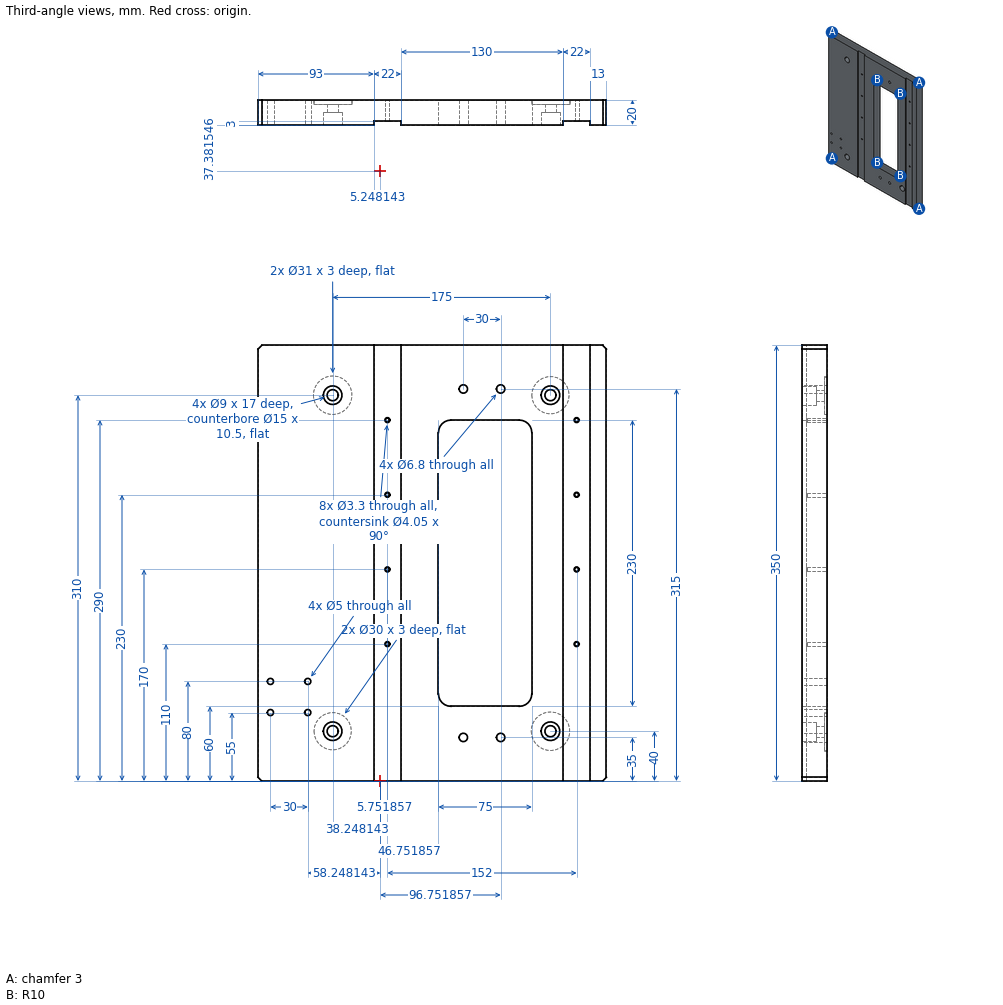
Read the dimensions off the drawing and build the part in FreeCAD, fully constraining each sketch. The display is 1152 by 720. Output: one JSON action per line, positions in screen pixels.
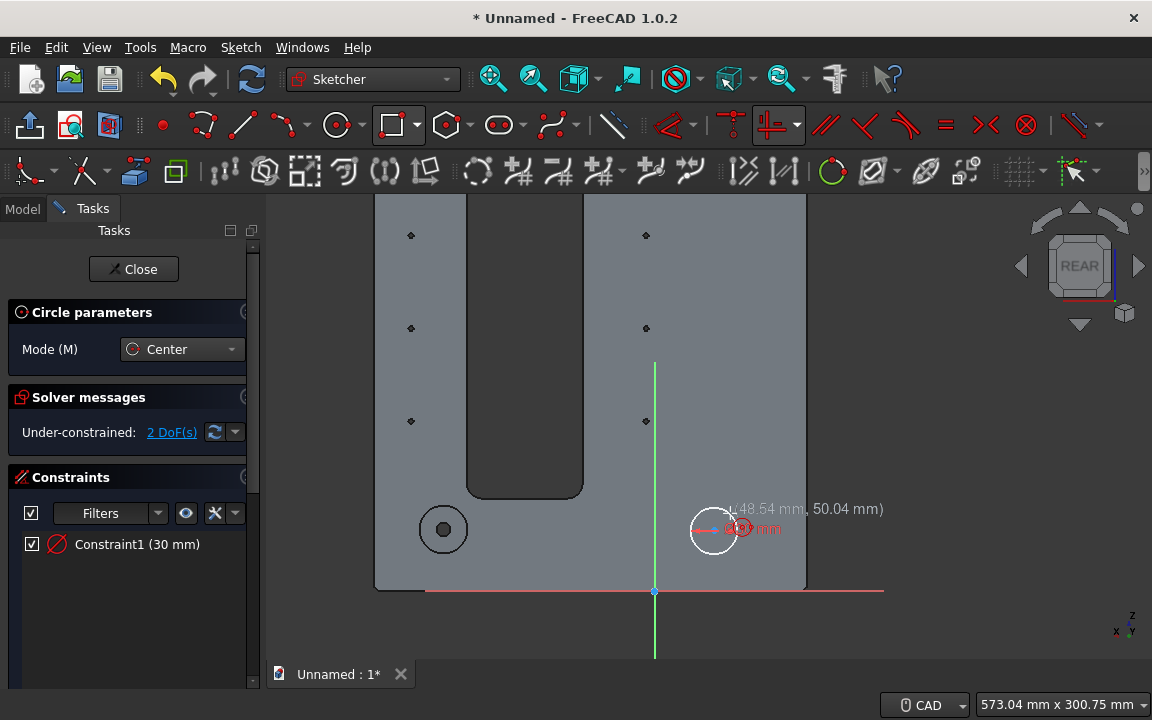
{"action": "scroll", "coordinate": [716, 532], "scroll_direction": "down", "scroll_amount": 3}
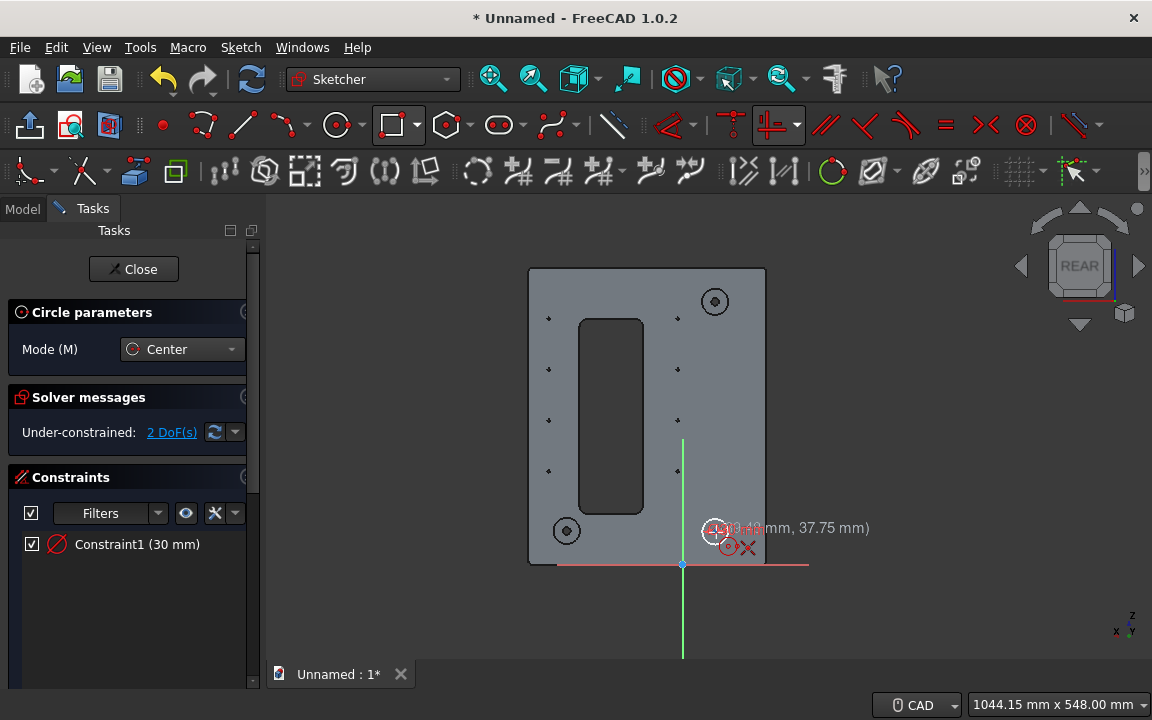
{"action": "scroll", "coordinate": [567, 302], "scroll_direction": "up", "scroll_amount": 3}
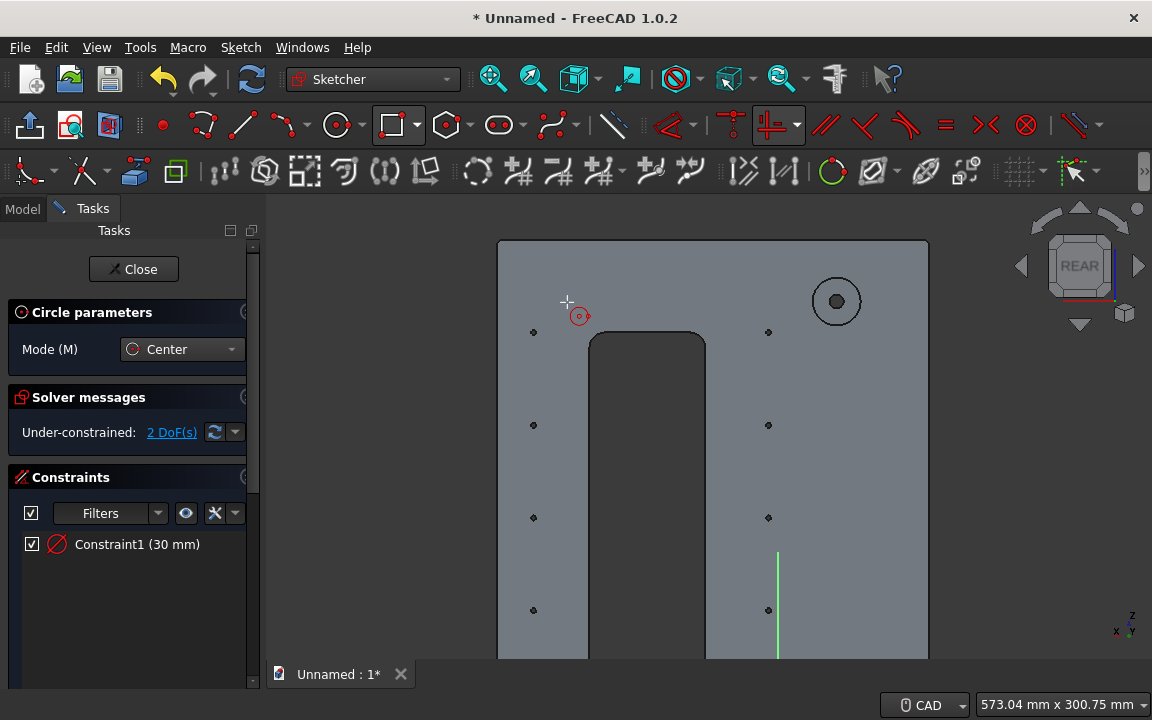
{"action": "left_click", "coordinate": [566, 302]}
{"action": "mouse_move", "coordinate": [583, 285]}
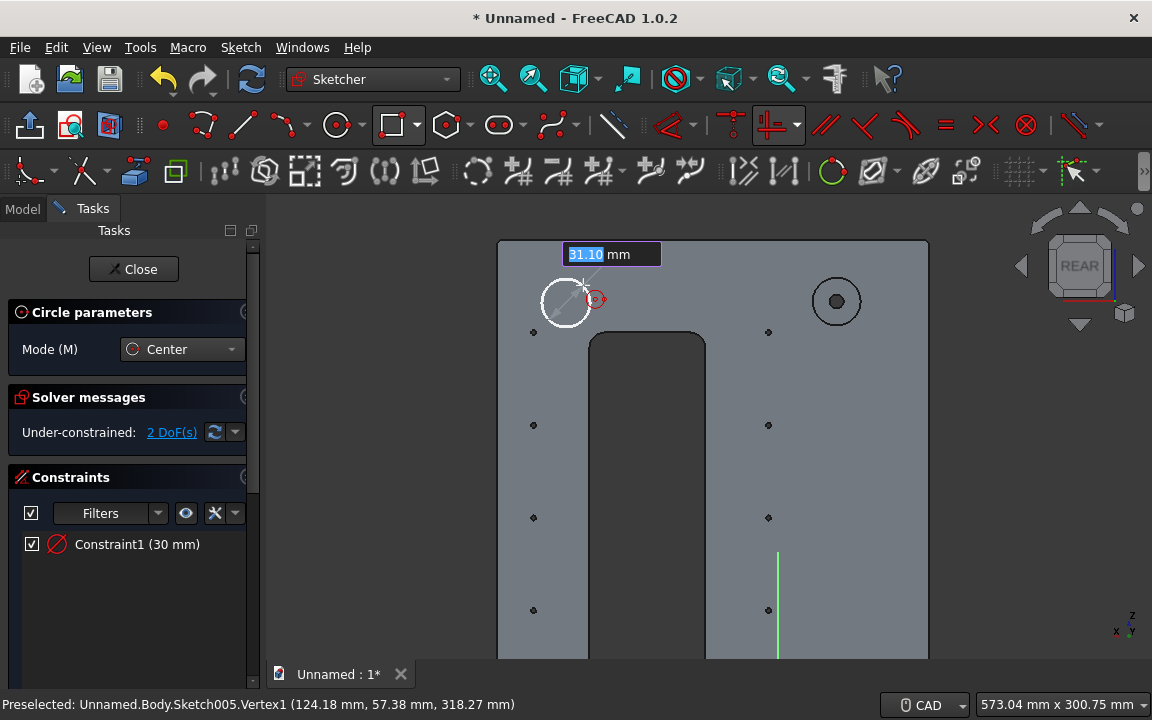
{"action": "type", "text": "30"}
{"action": "key", "text": "Return"}
{"action": "key", "text": "Escape"}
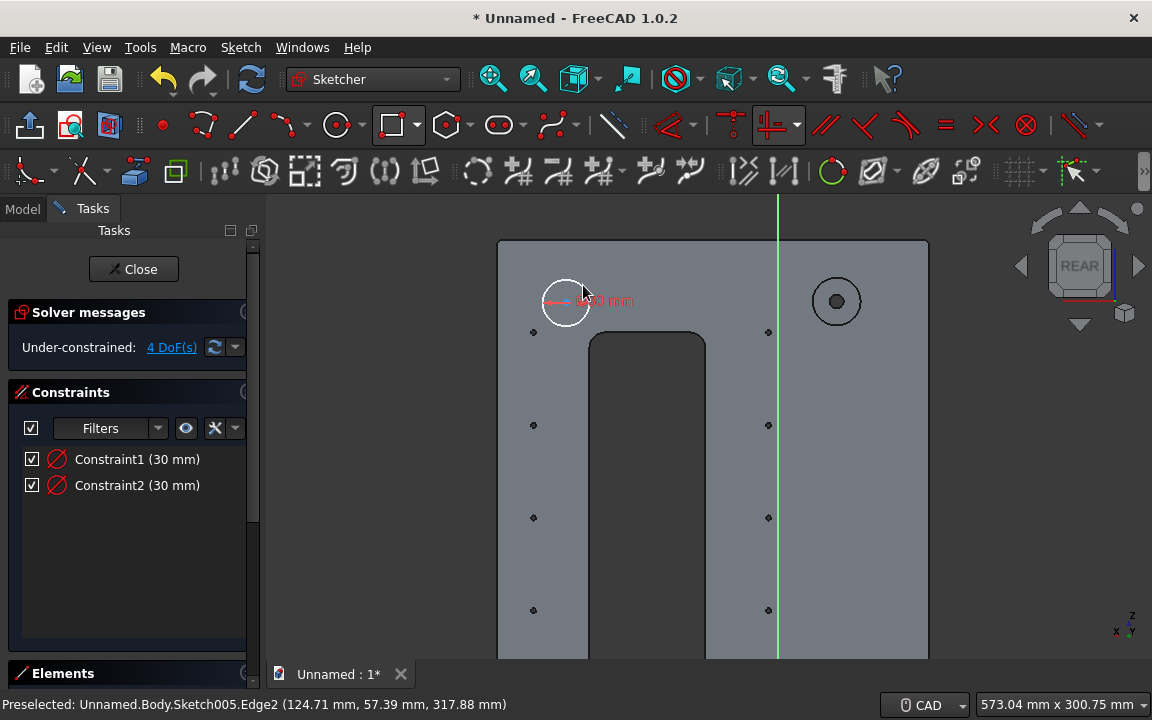
{"action": "left_click", "coordinate": [668, 126]}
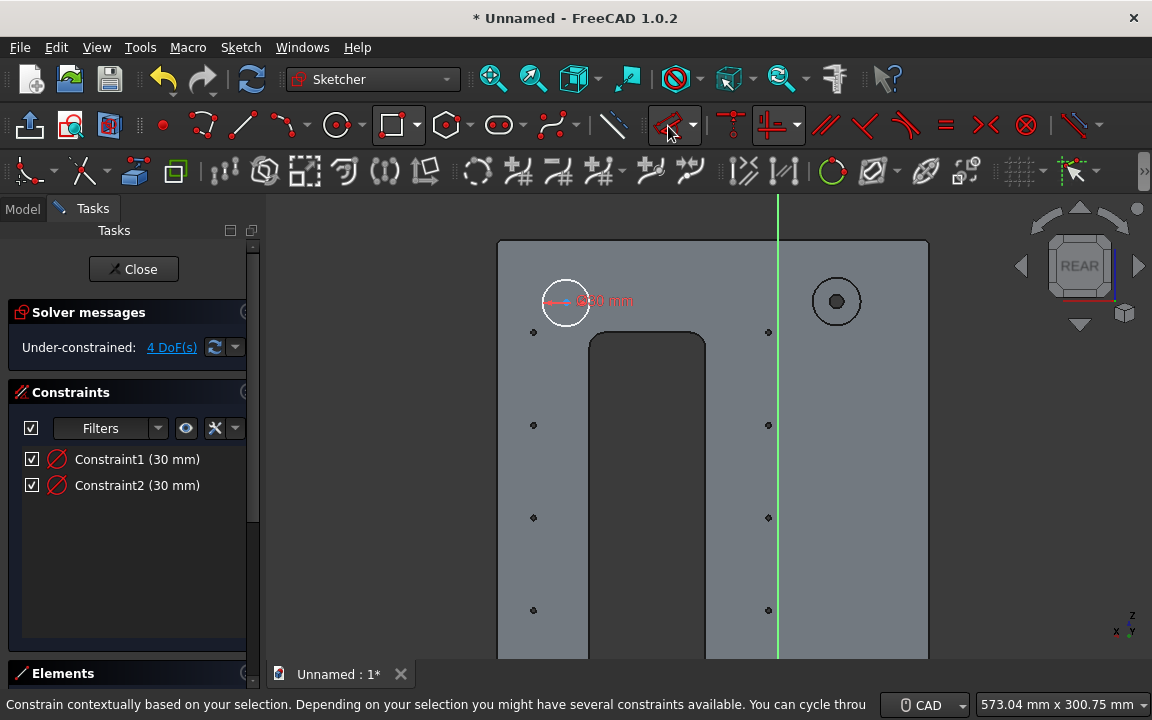
{"action": "scroll", "coordinate": [566, 301], "scroll_direction": "down", "scroll_amount": 3}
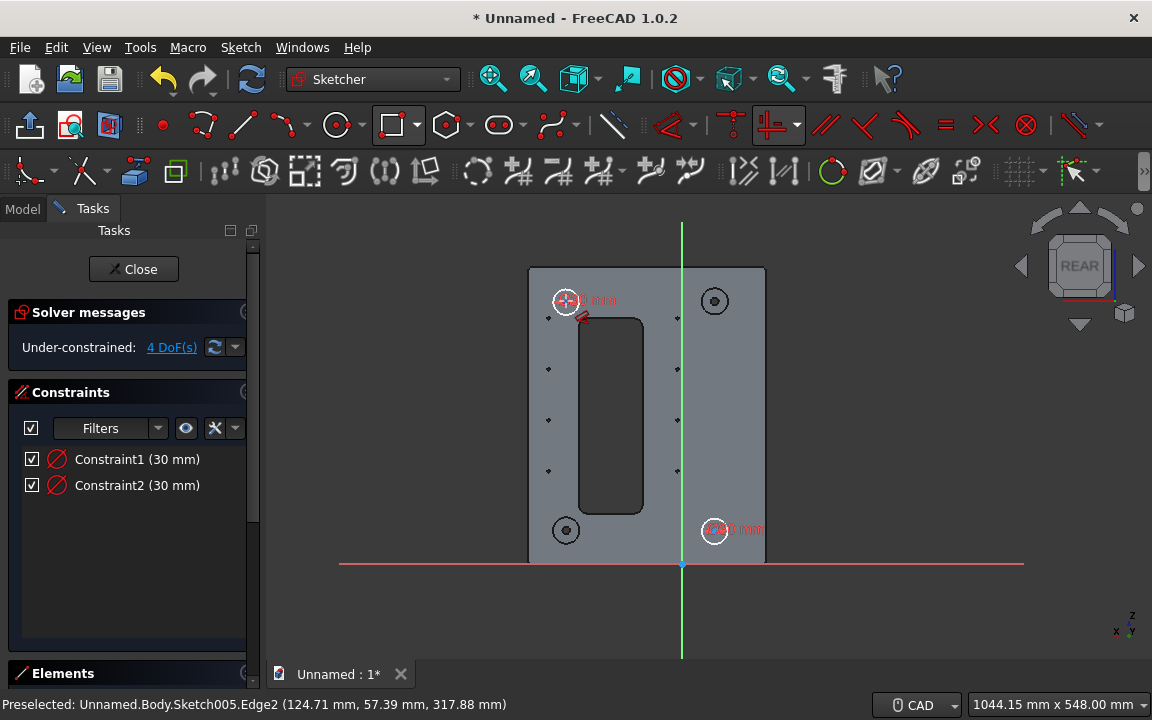
{"action": "left_click", "coordinate": [715, 531]}
{"action": "left_click", "coordinate": [749, 548]}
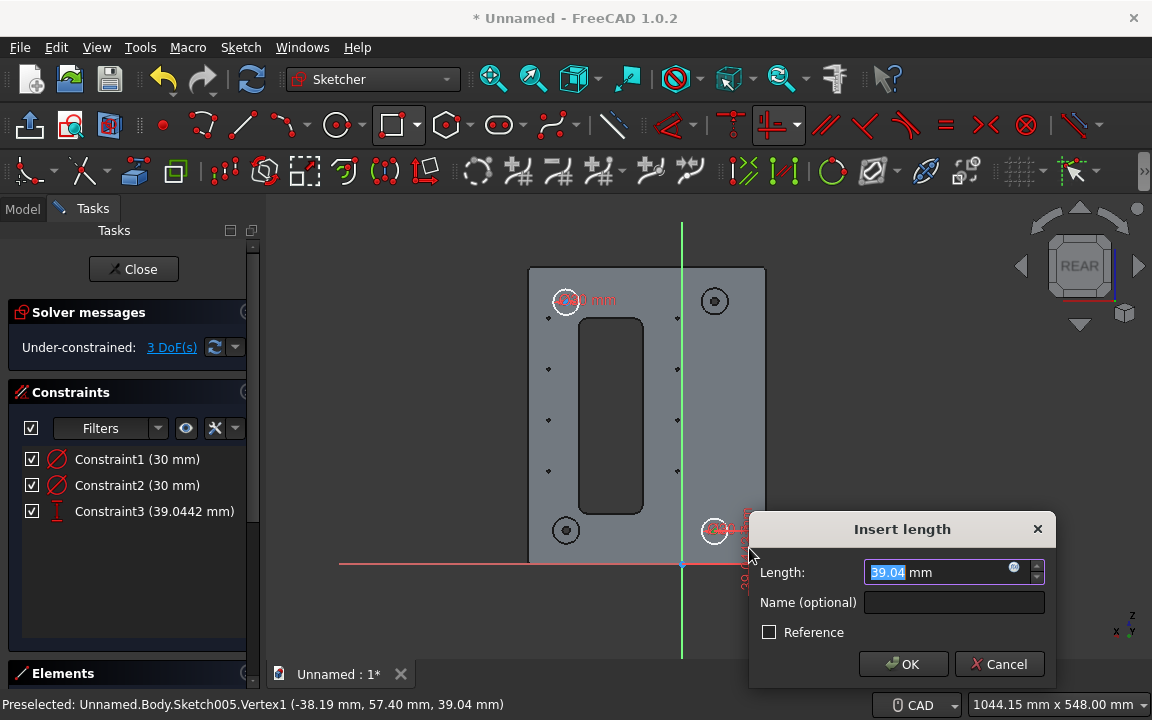
{"action": "type", "text": "40"}
{"action": "key", "text": "Return"}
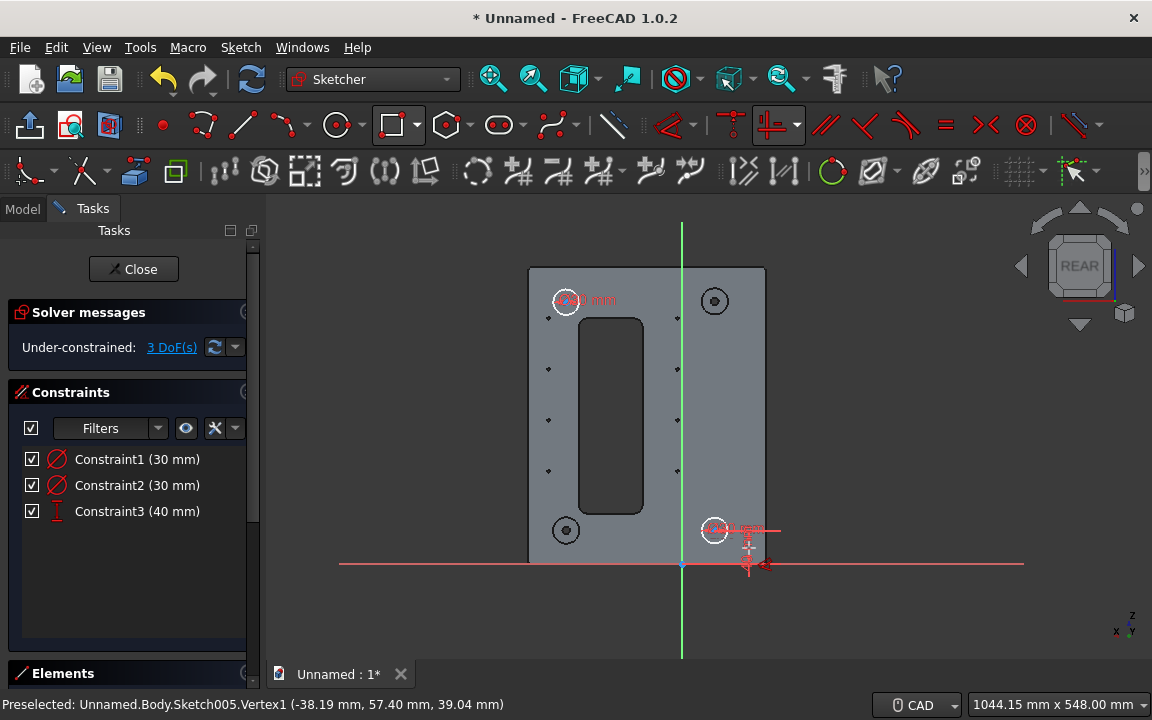
{"action": "left_click", "coordinate": [566, 302]}
{"action": "left_click", "coordinate": [532, 433]}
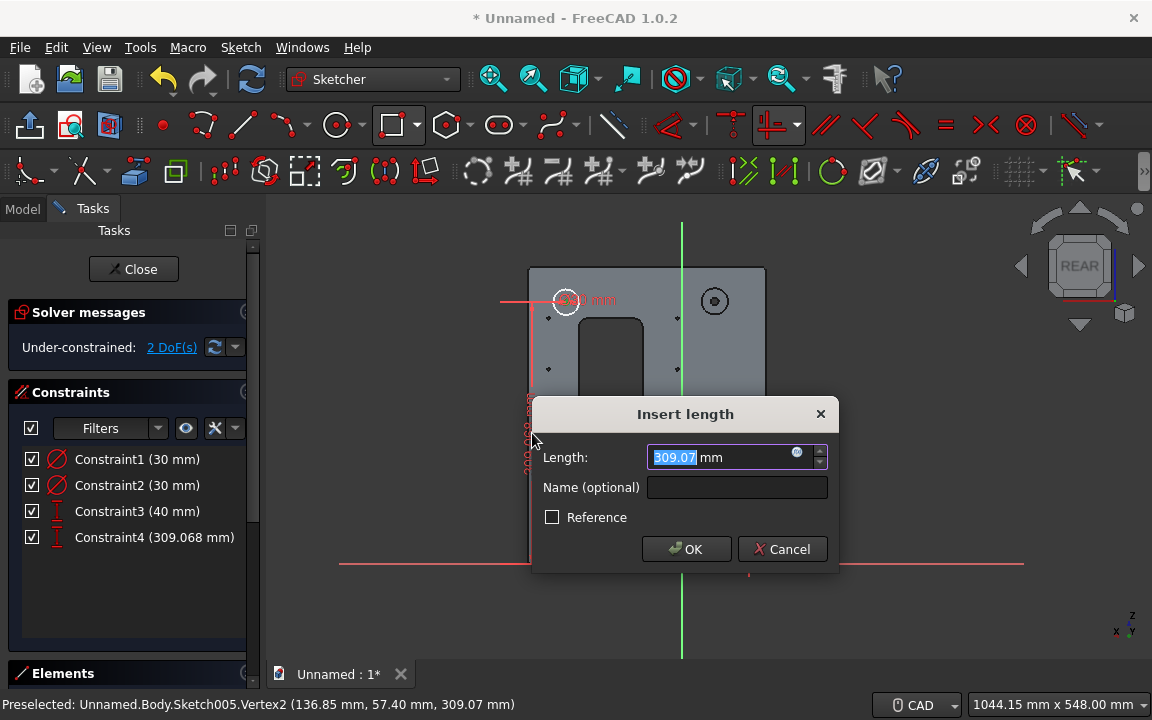
{"action": "type", "text": "310"}
{"action": "key", "text": "Return"}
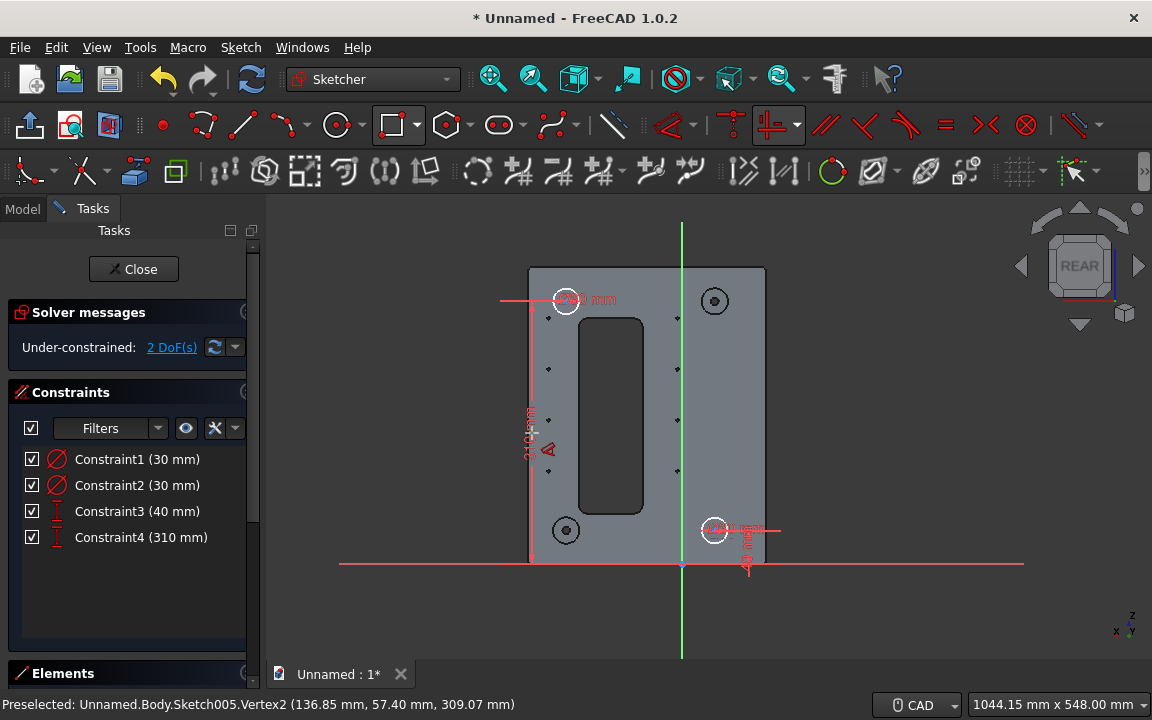
{"action": "left_click", "coordinate": [715, 531]}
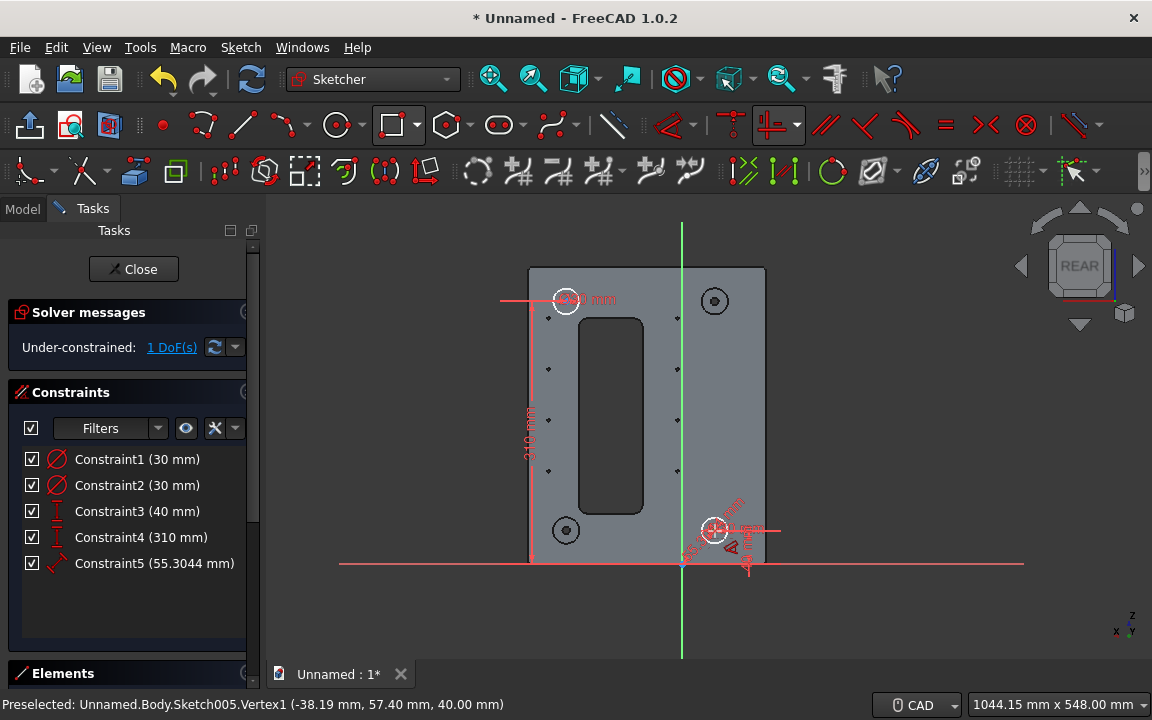
{"action": "left_click", "coordinate": [566, 301]}
{"action": "left_click", "coordinate": [640, 267]}